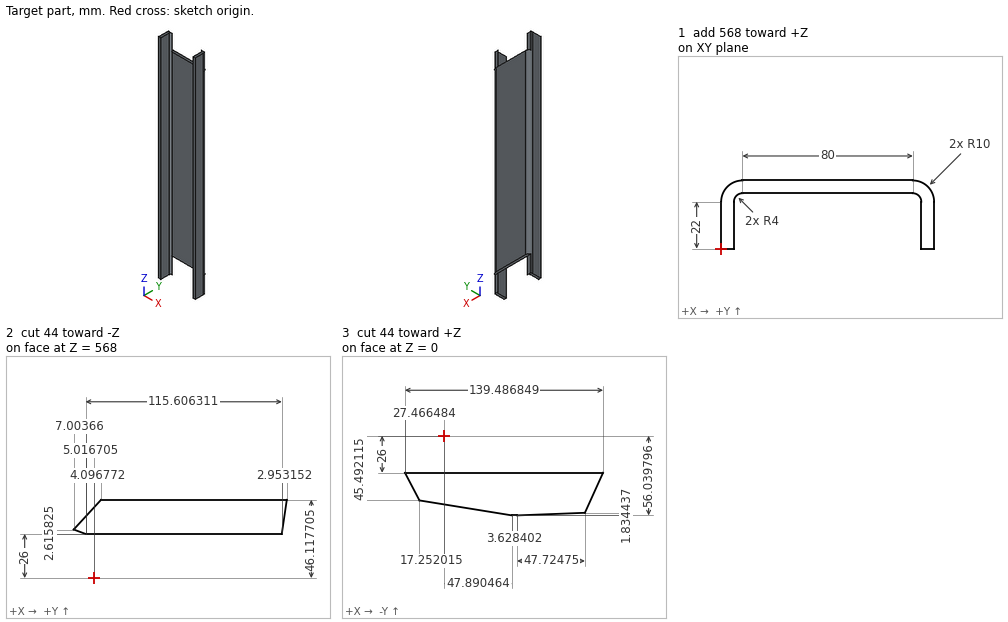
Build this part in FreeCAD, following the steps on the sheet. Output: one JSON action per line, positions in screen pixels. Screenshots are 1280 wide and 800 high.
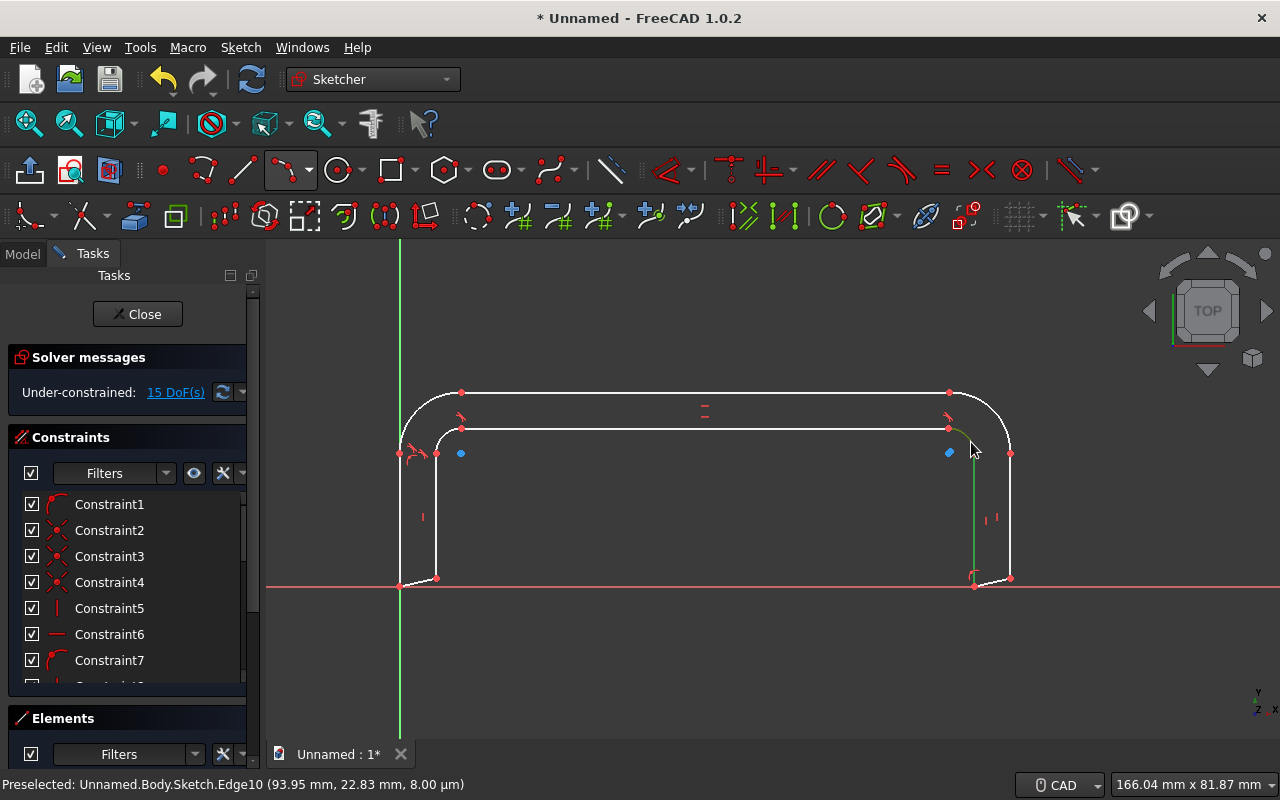
{"action": "key", "text": "t"}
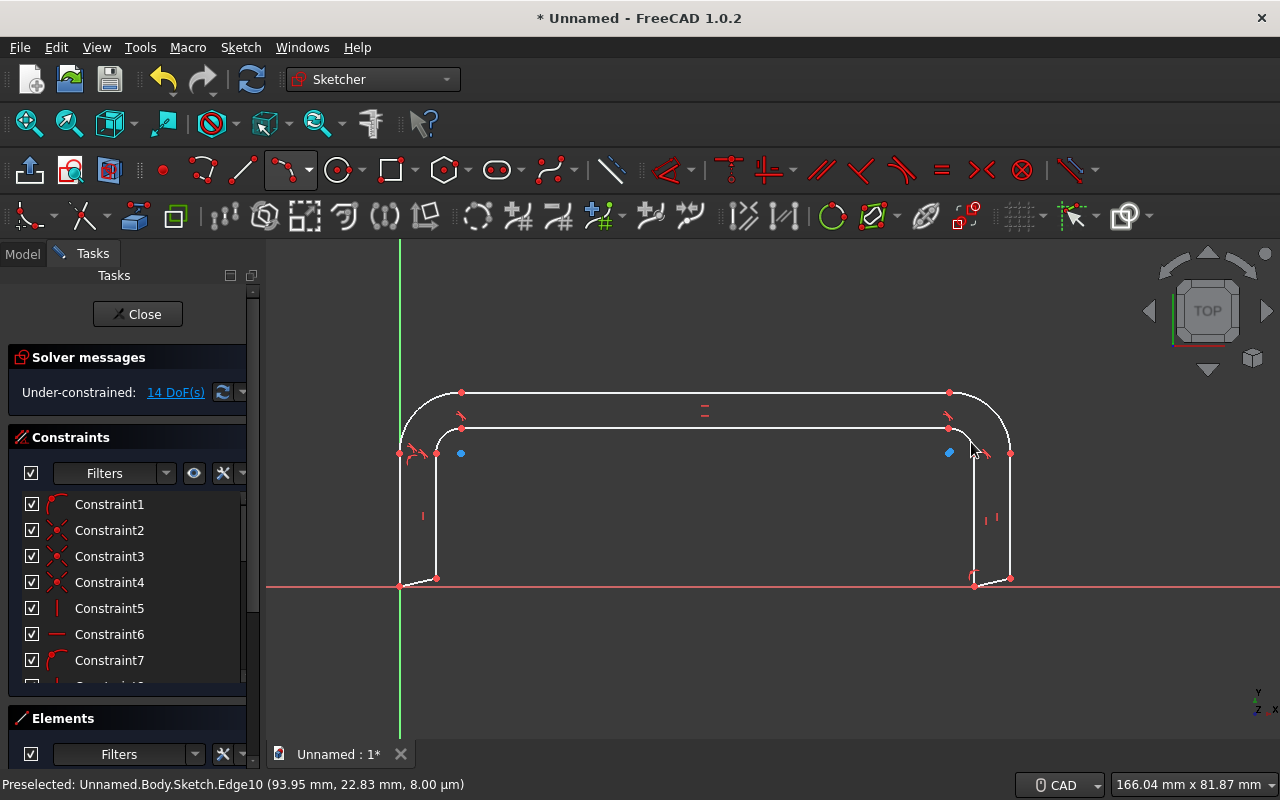
{"action": "left_click", "coordinate": [1010, 541]}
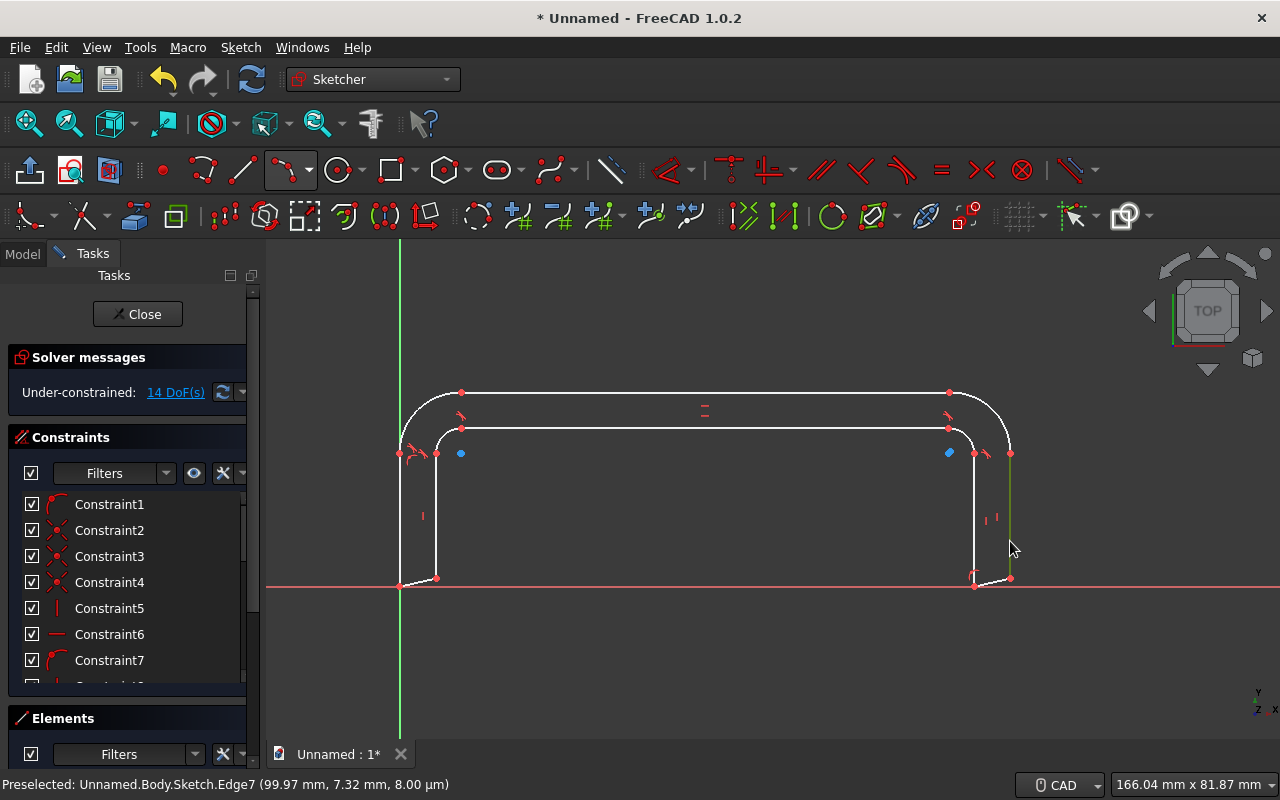
{"action": "left_click", "coordinate": [1004, 425]}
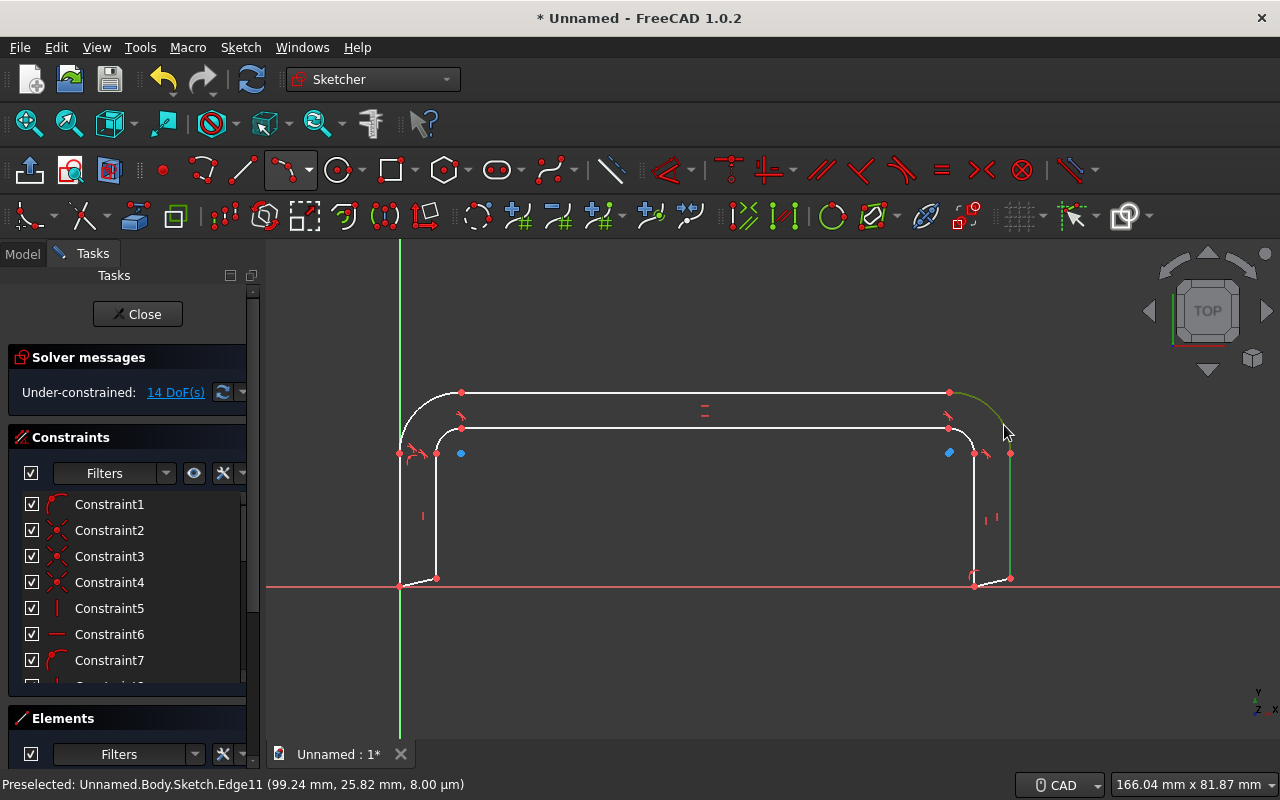
{"action": "key", "text": "t"}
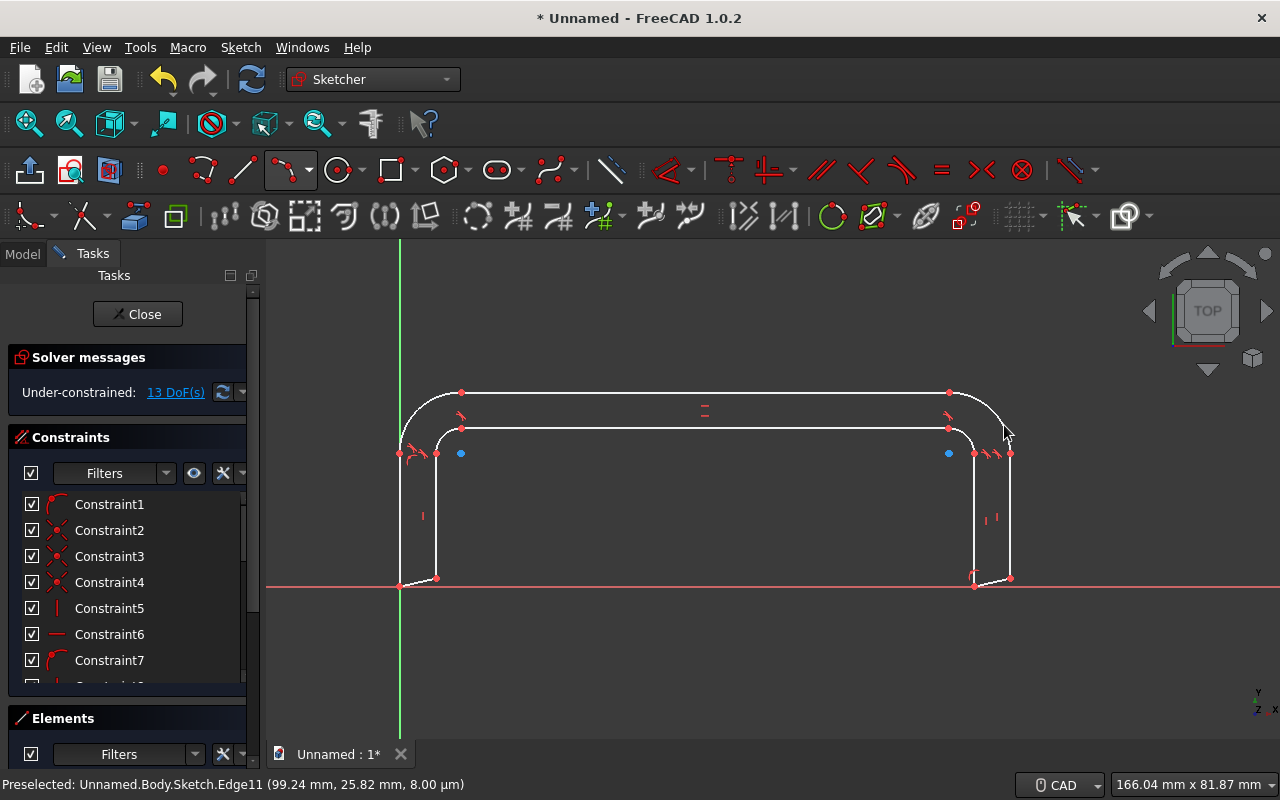
{"action": "left_click", "coordinate": [803, 393]}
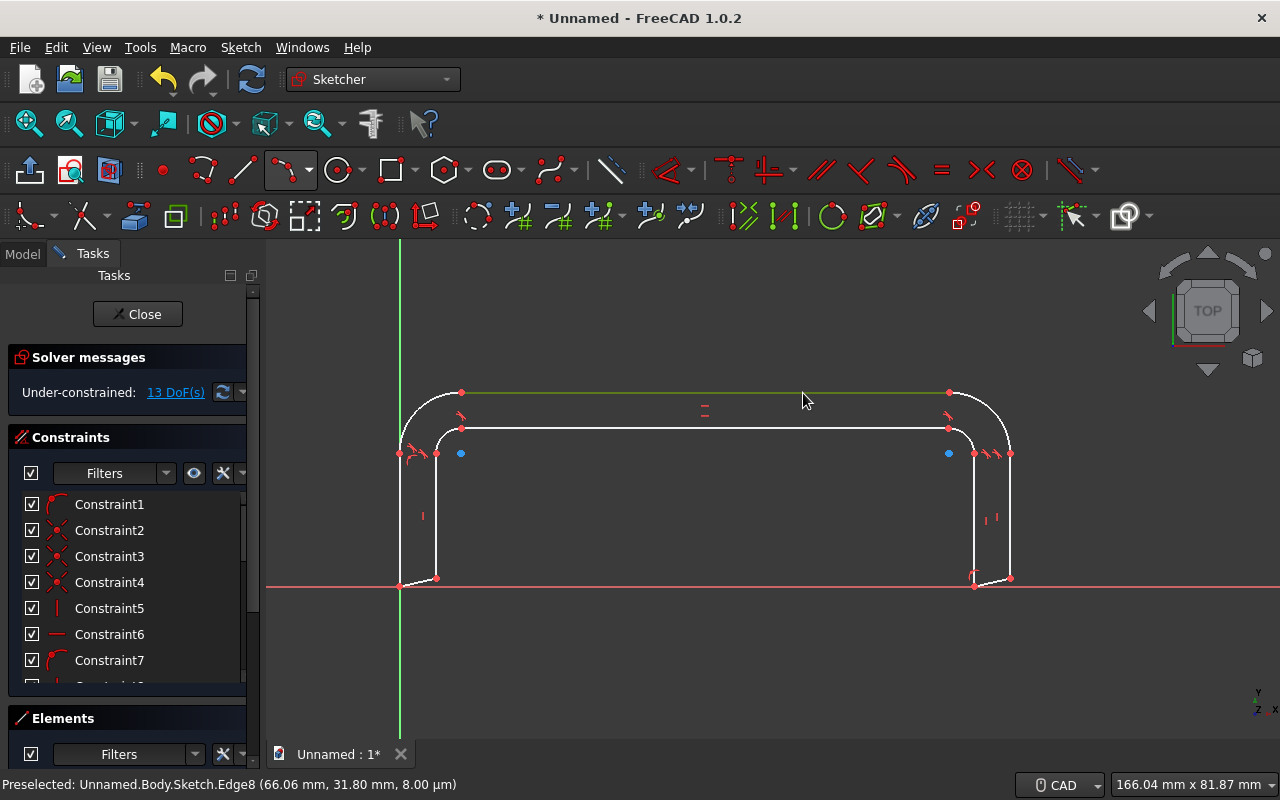
{"action": "left_click", "coordinate": [1003, 426]}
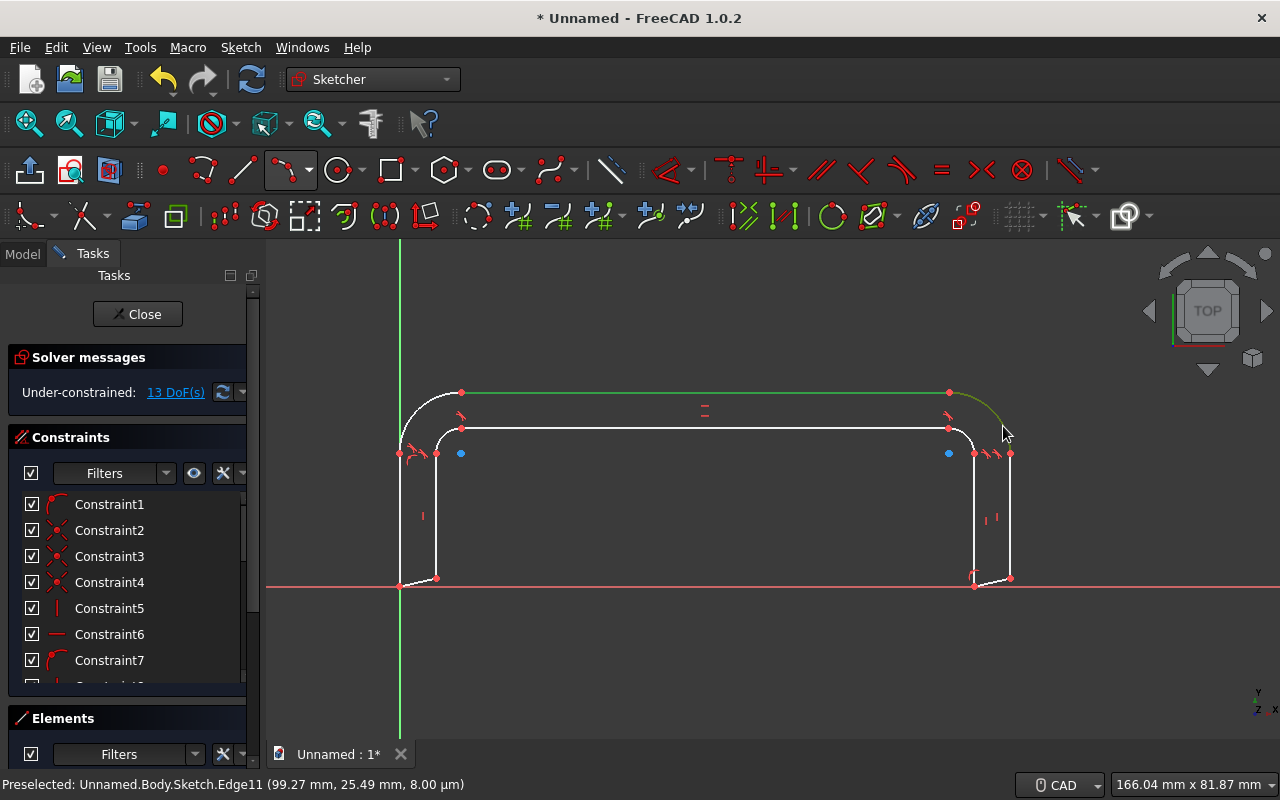
{"action": "left_click", "coordinate": [902, 170]}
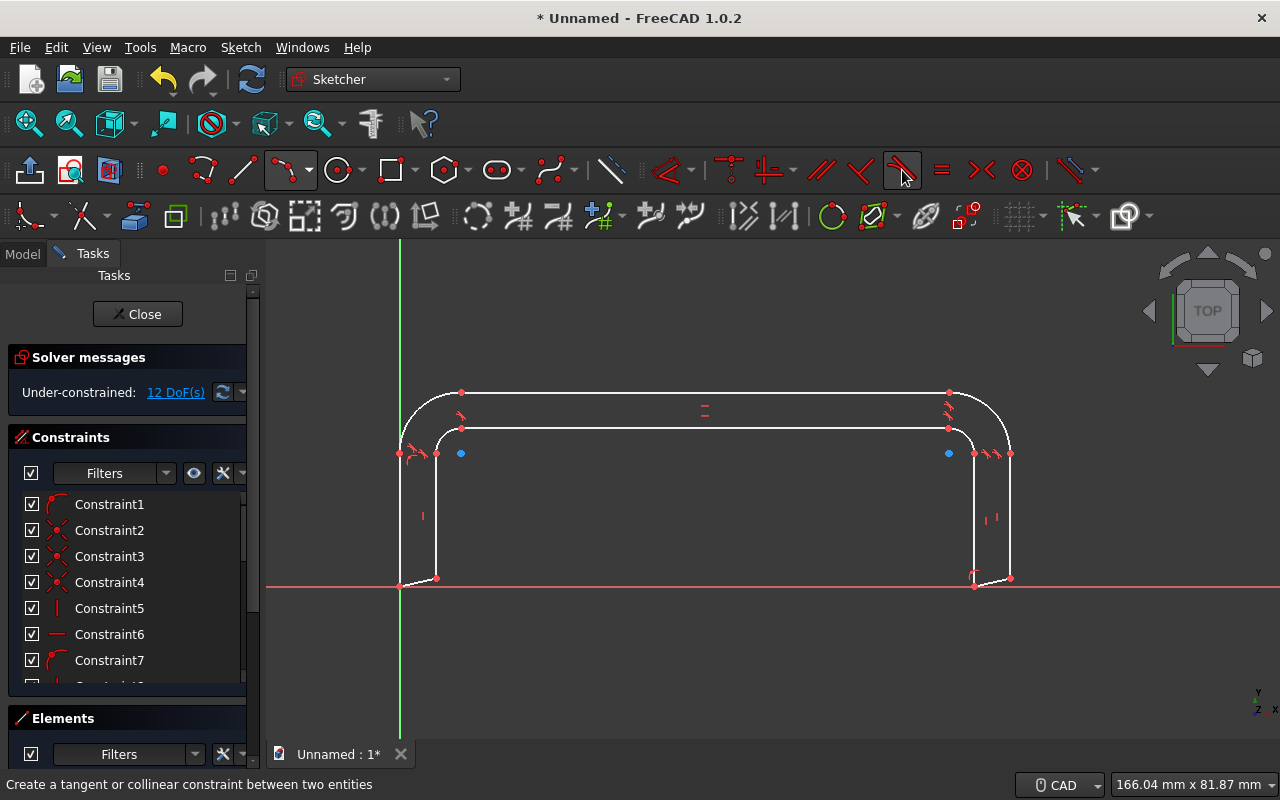
{"action": "left_click", "coordinate": [803, 393]}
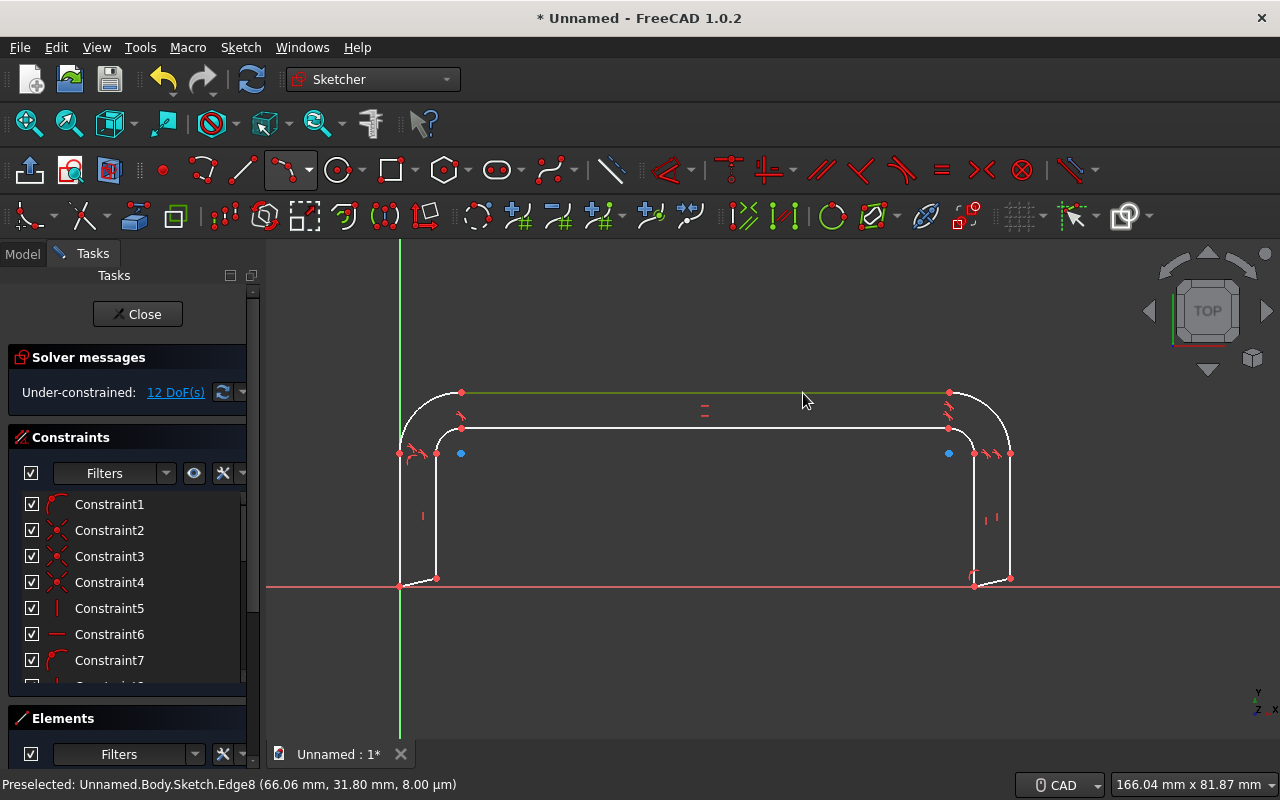
{"action": "left_click", "coordinate": [433, 399]}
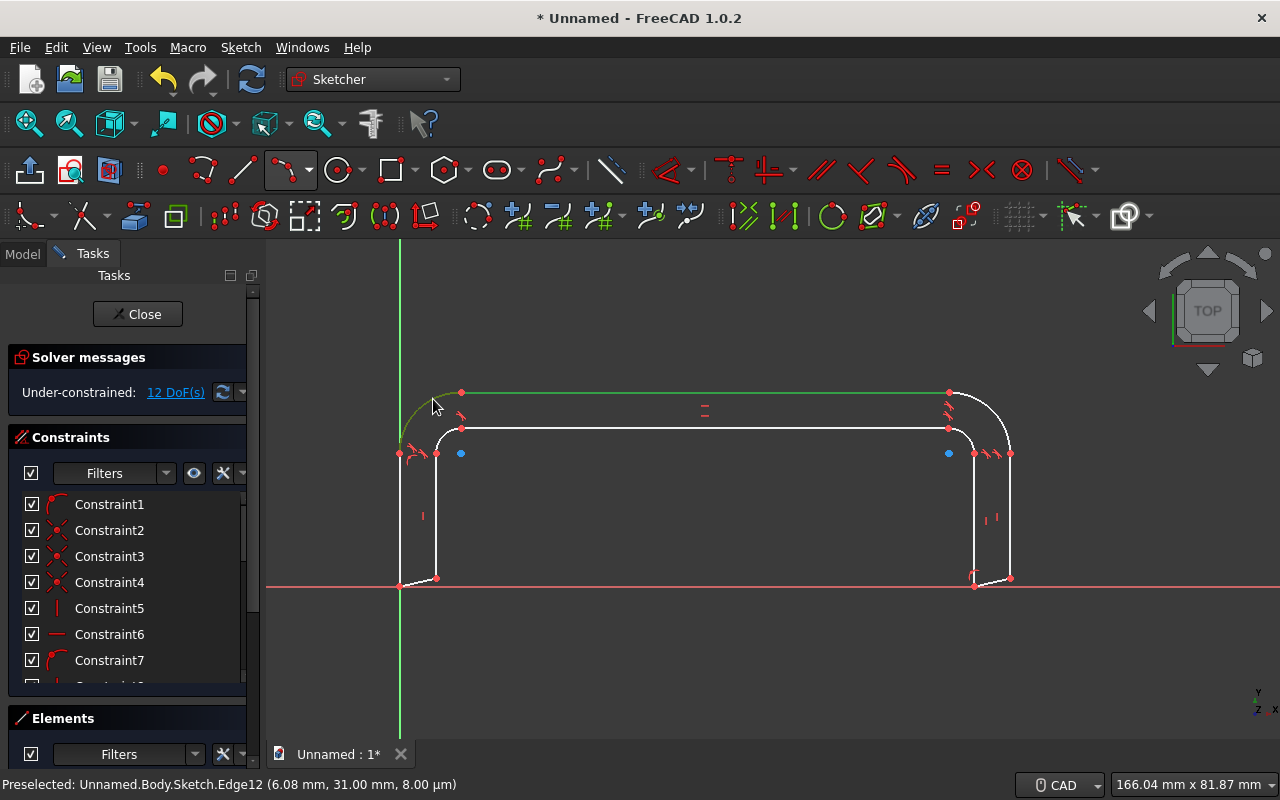
{"action": "left_click", "coordinate": [902, 170]}